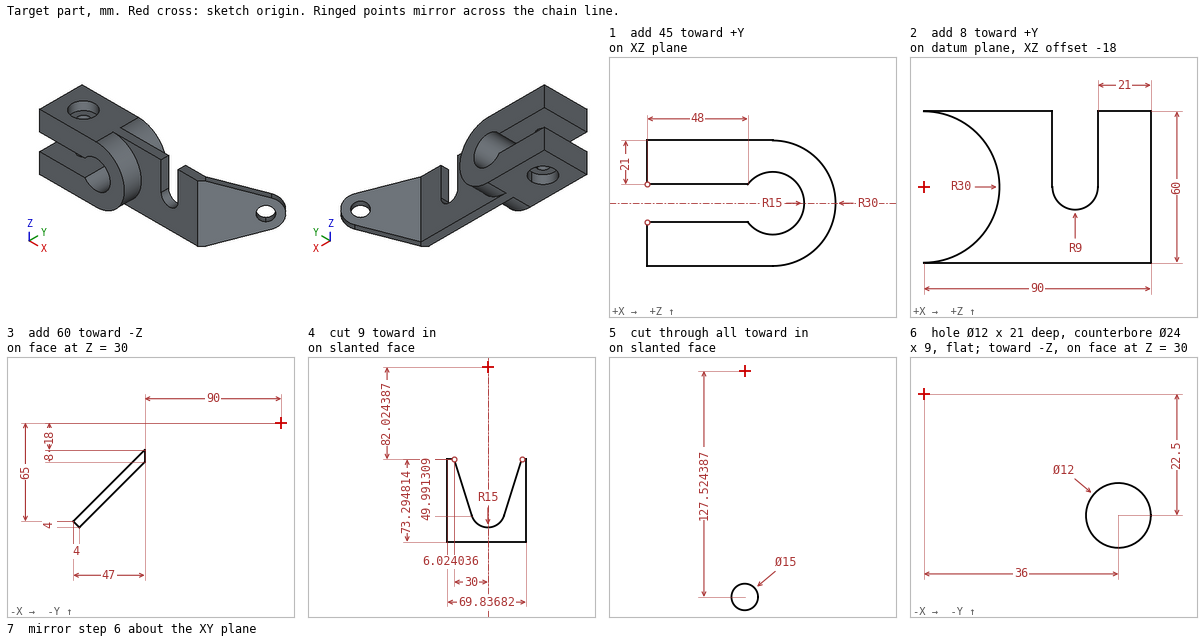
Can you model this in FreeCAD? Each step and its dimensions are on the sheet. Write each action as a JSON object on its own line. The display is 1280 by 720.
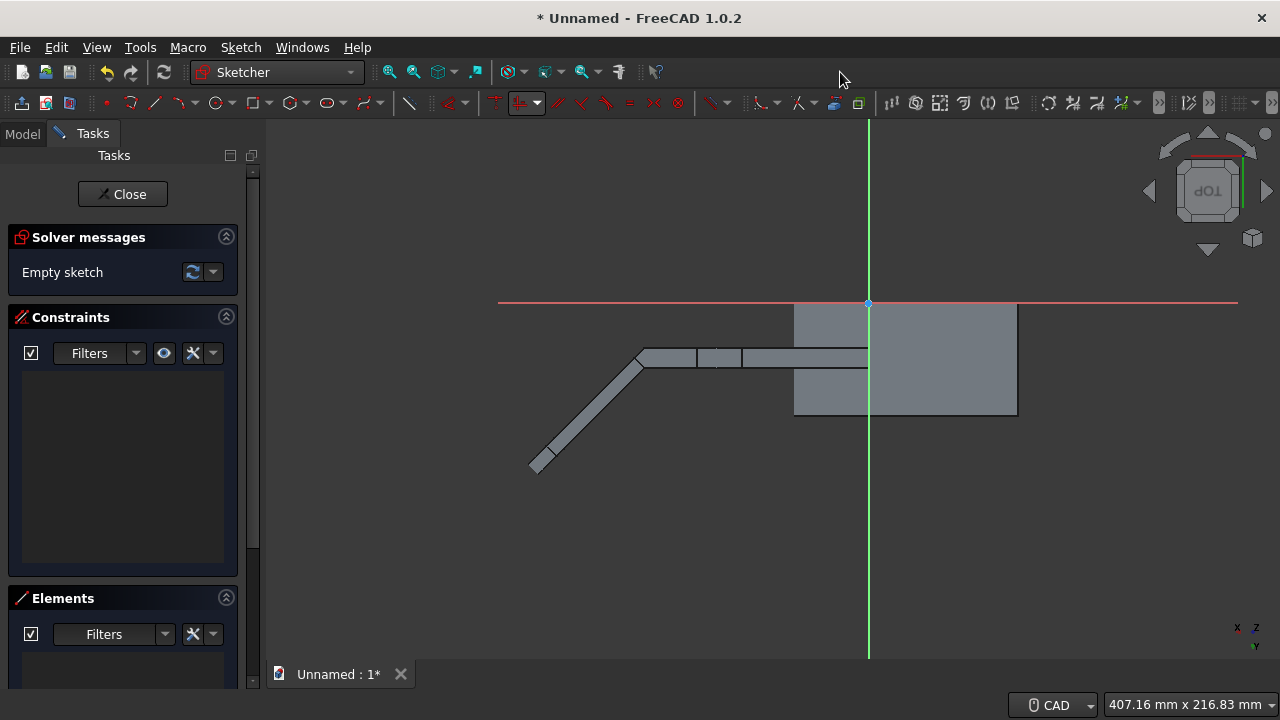
{"action": "scroll", "coordinate": [983, 357], "scroll_direction": "up", "scroll_amount": 12}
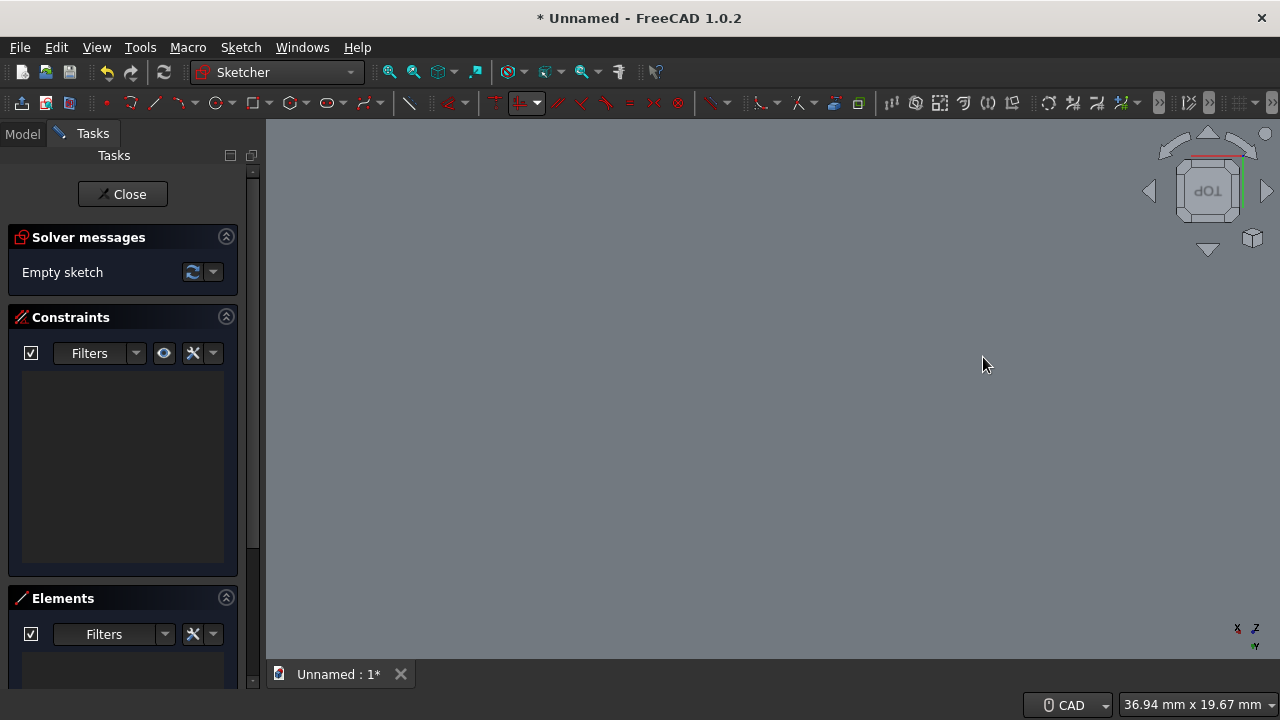
{"action": "left_click", "coordinate": [216, 104]}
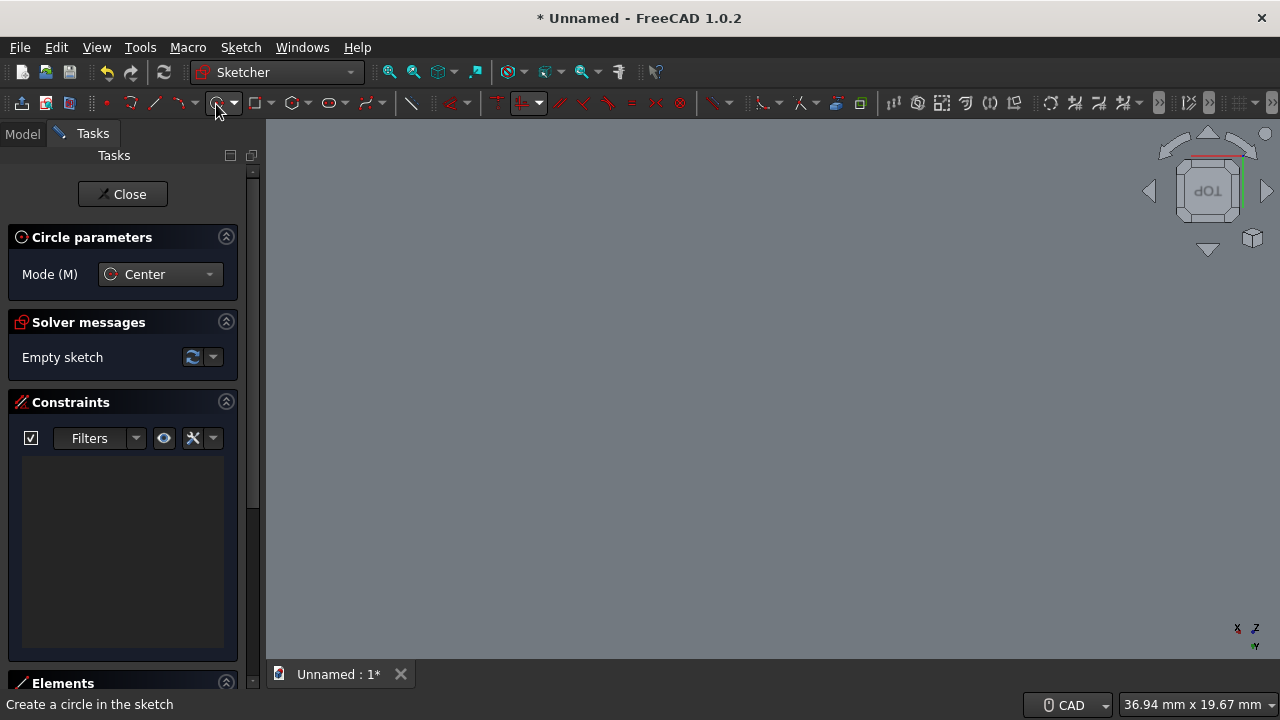
{"action": "left_click", "coordinate": [702, 380]}
{"action": "mouse_move", "coordinate": [819, 263]}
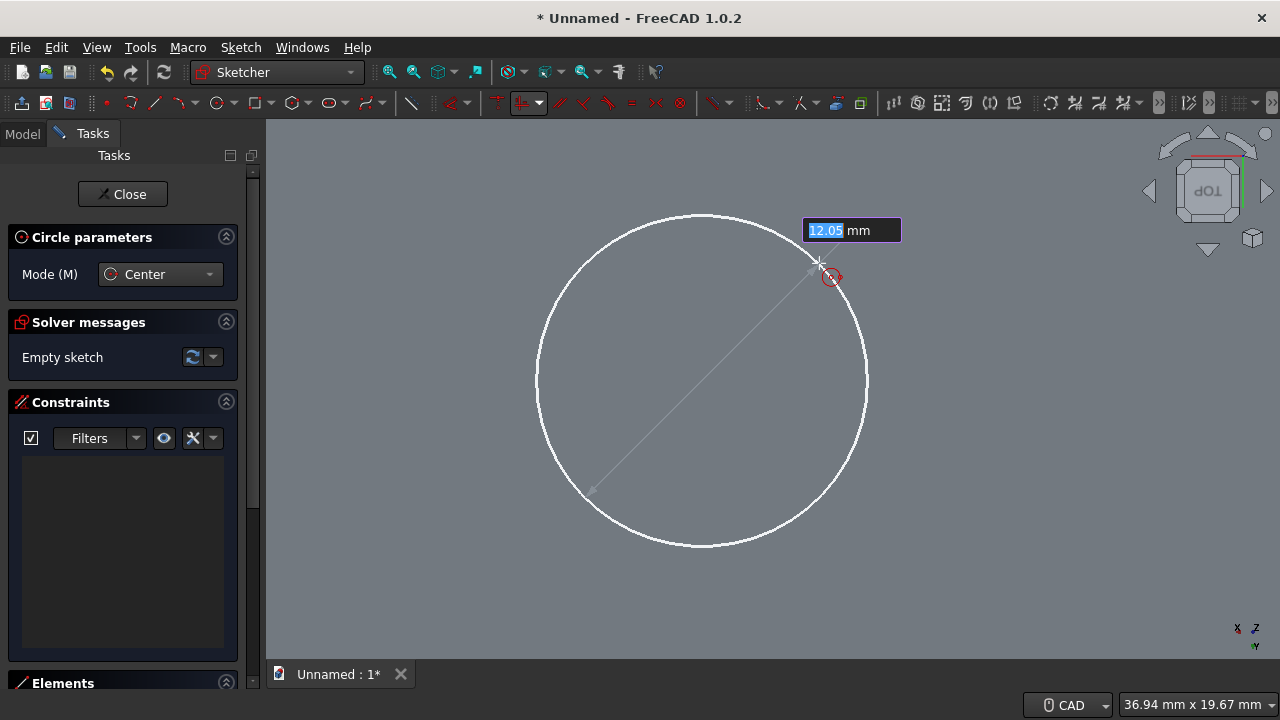
{"action": "type", "text": "12"}
{"action": "key", "text": "Return"}
{"action": "key", "text": "Escape"}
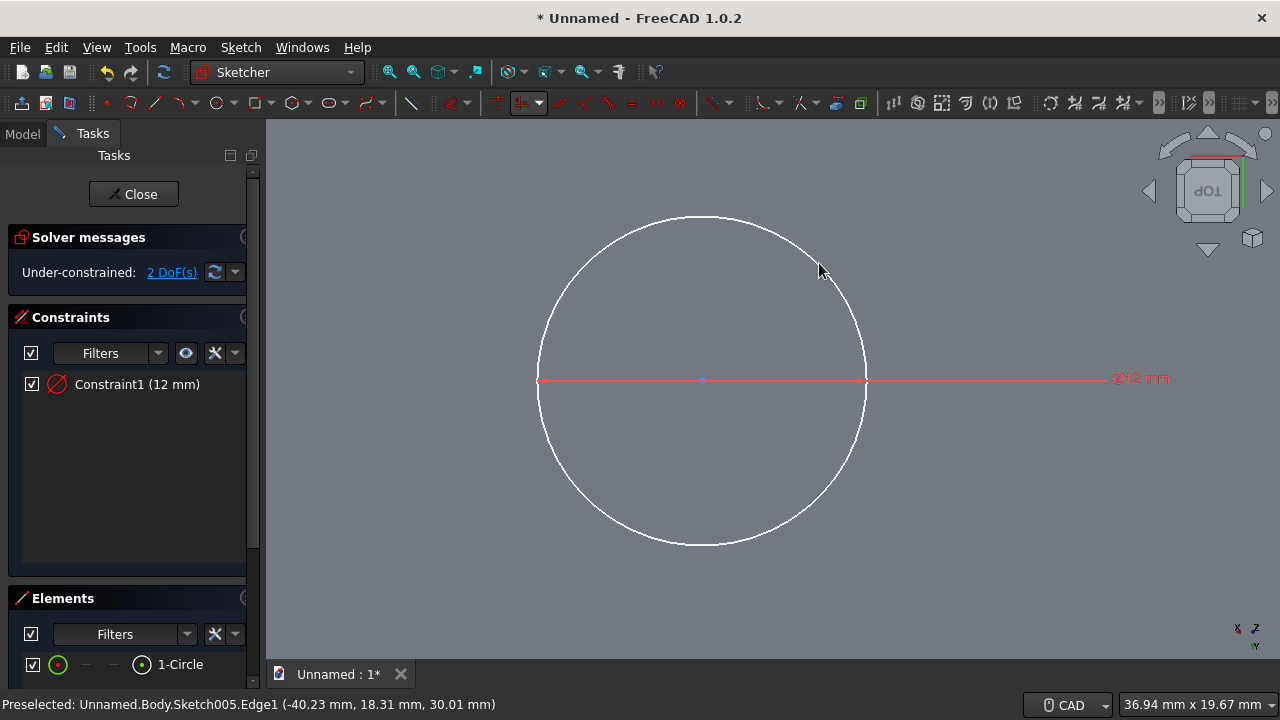
{"action": "left_click", "coordinate": [450, 104]}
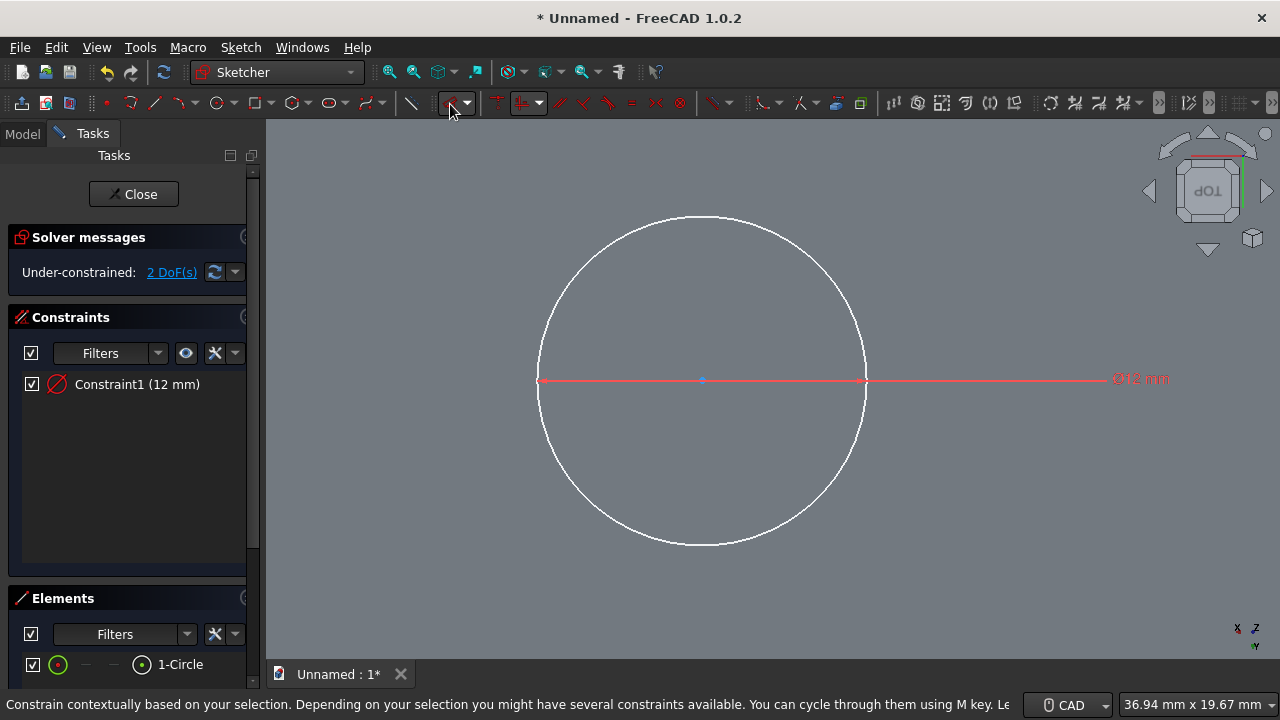
{"action": "left_click", "coordinate": [702, 381]}
{"action": "left_click", "coordinate": [498, 415]}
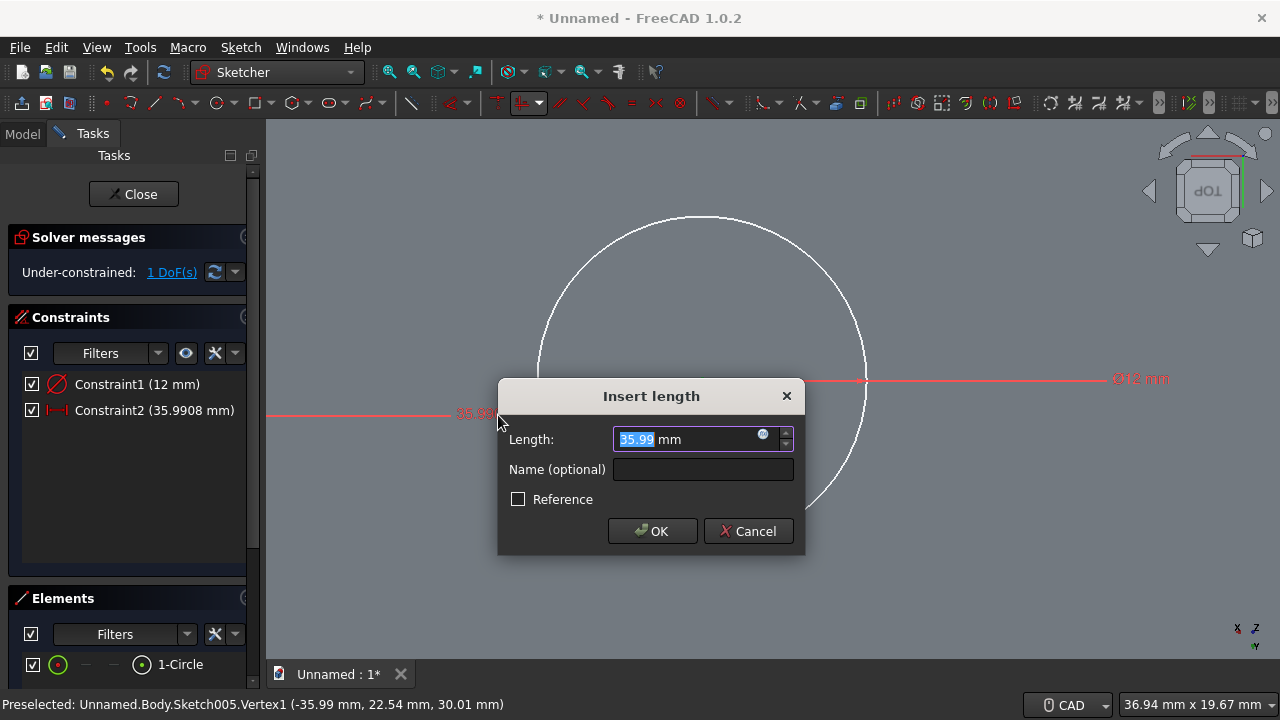
{"action": "type", "text": "36"}
{"action": "key", "text": "Return"}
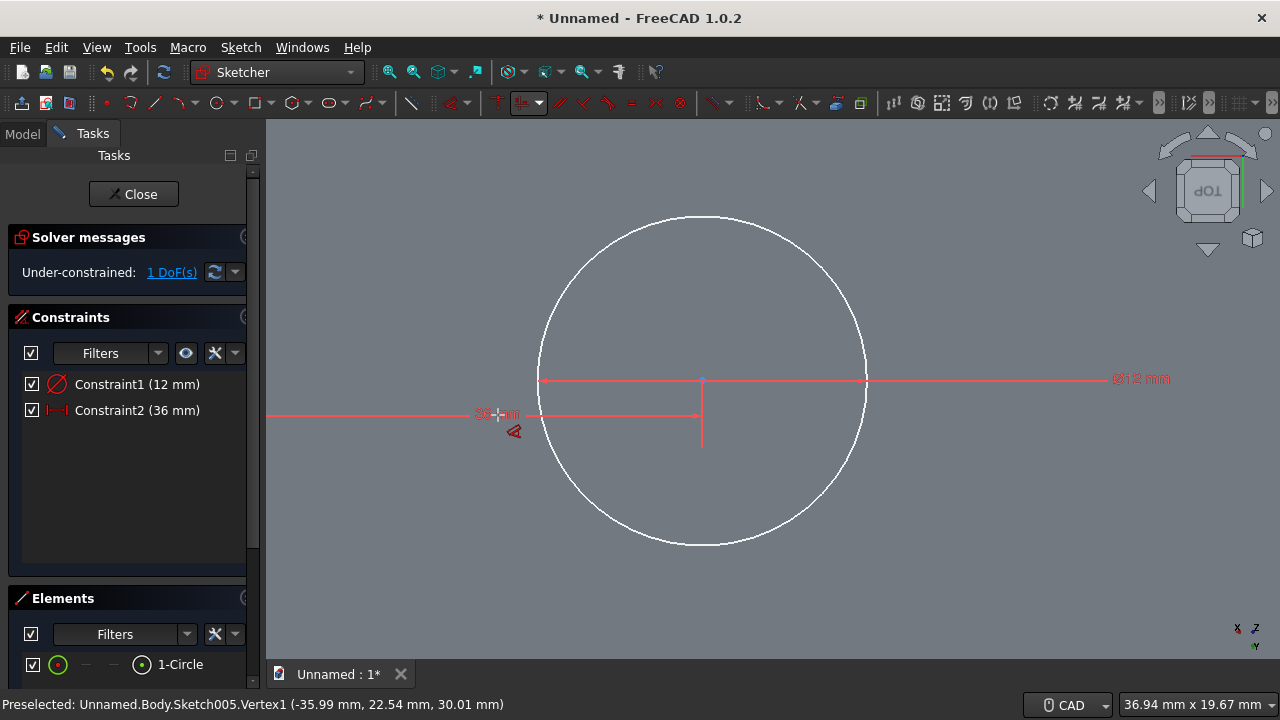
{"action": "left_click", "coordinate": [702, 381]}
{"action": "left_click", "coordinate": [736, 264]}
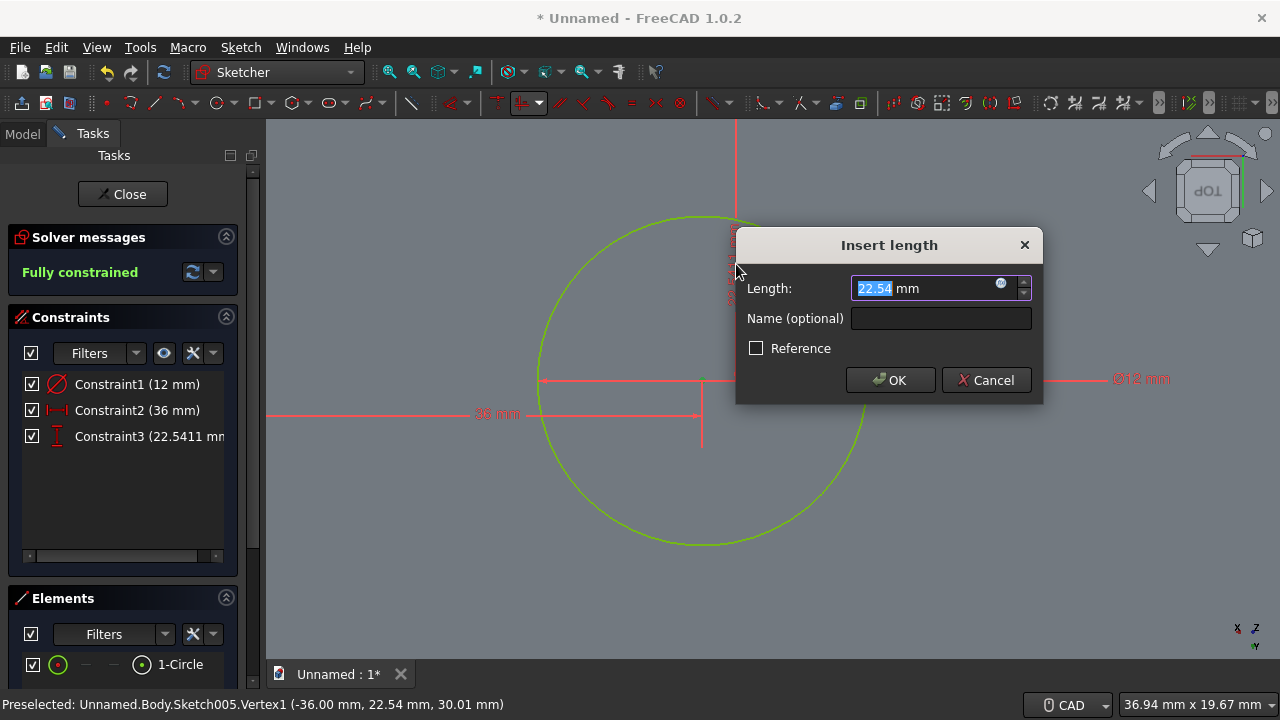
{"action": "type", "text": "22.5"}
{"action": "key", "text": "Return"}
{"action": "key", "text": "Escape"}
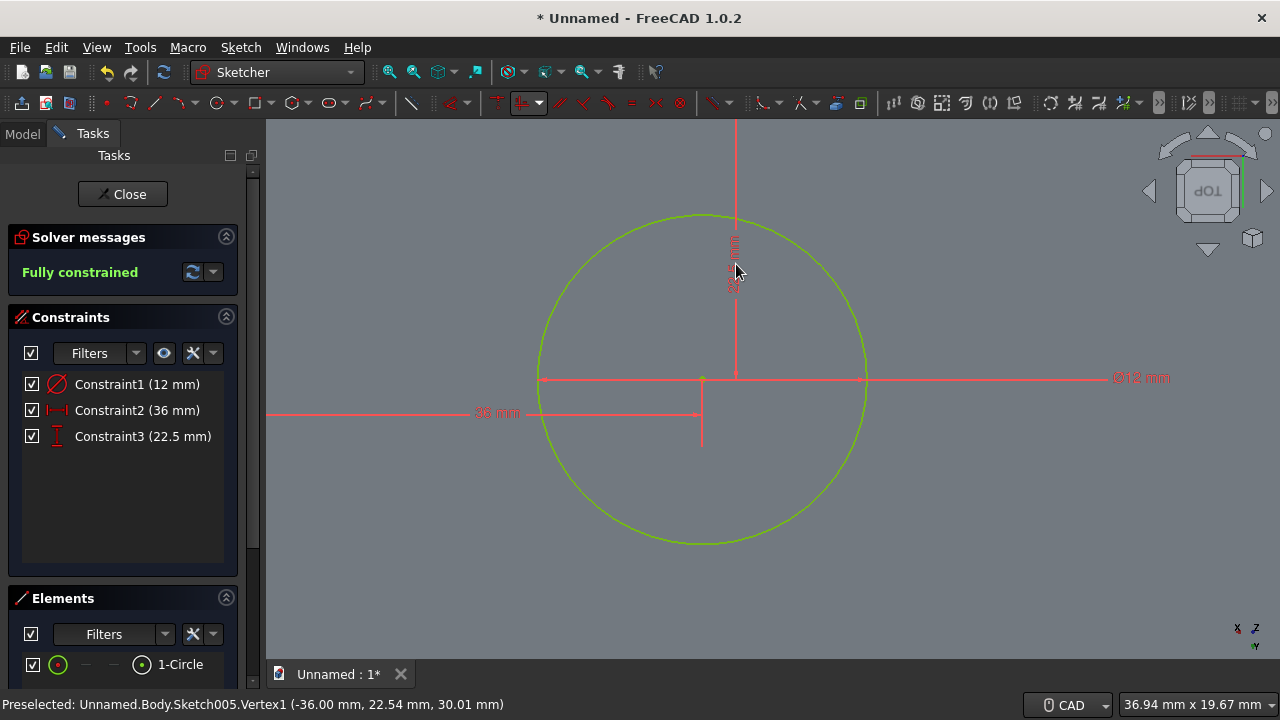
{"action": "left_click", "coordinate": [123, 194]}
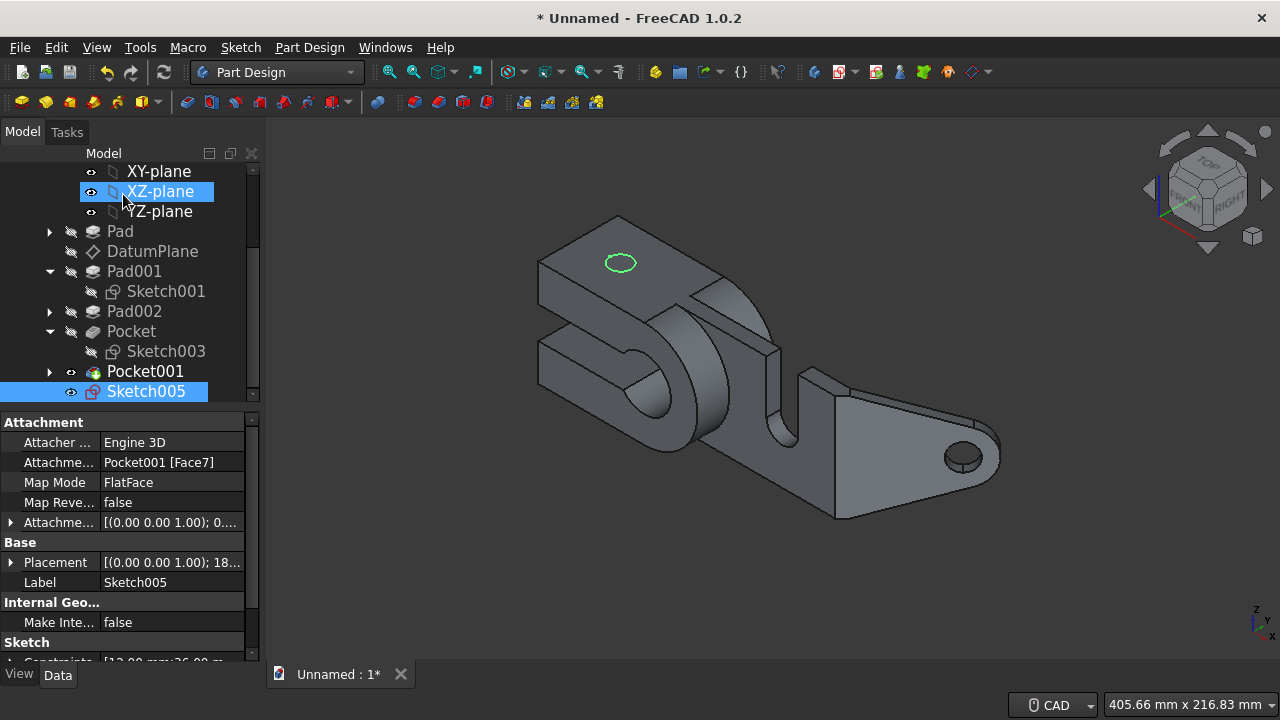
{"action": "left_click", "coordinate": [212, 102]}